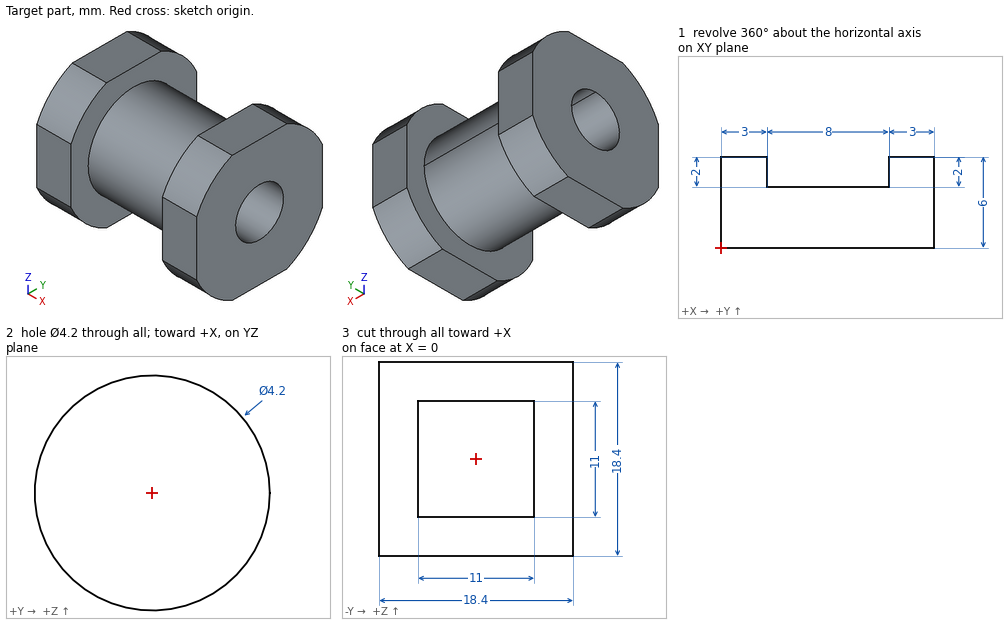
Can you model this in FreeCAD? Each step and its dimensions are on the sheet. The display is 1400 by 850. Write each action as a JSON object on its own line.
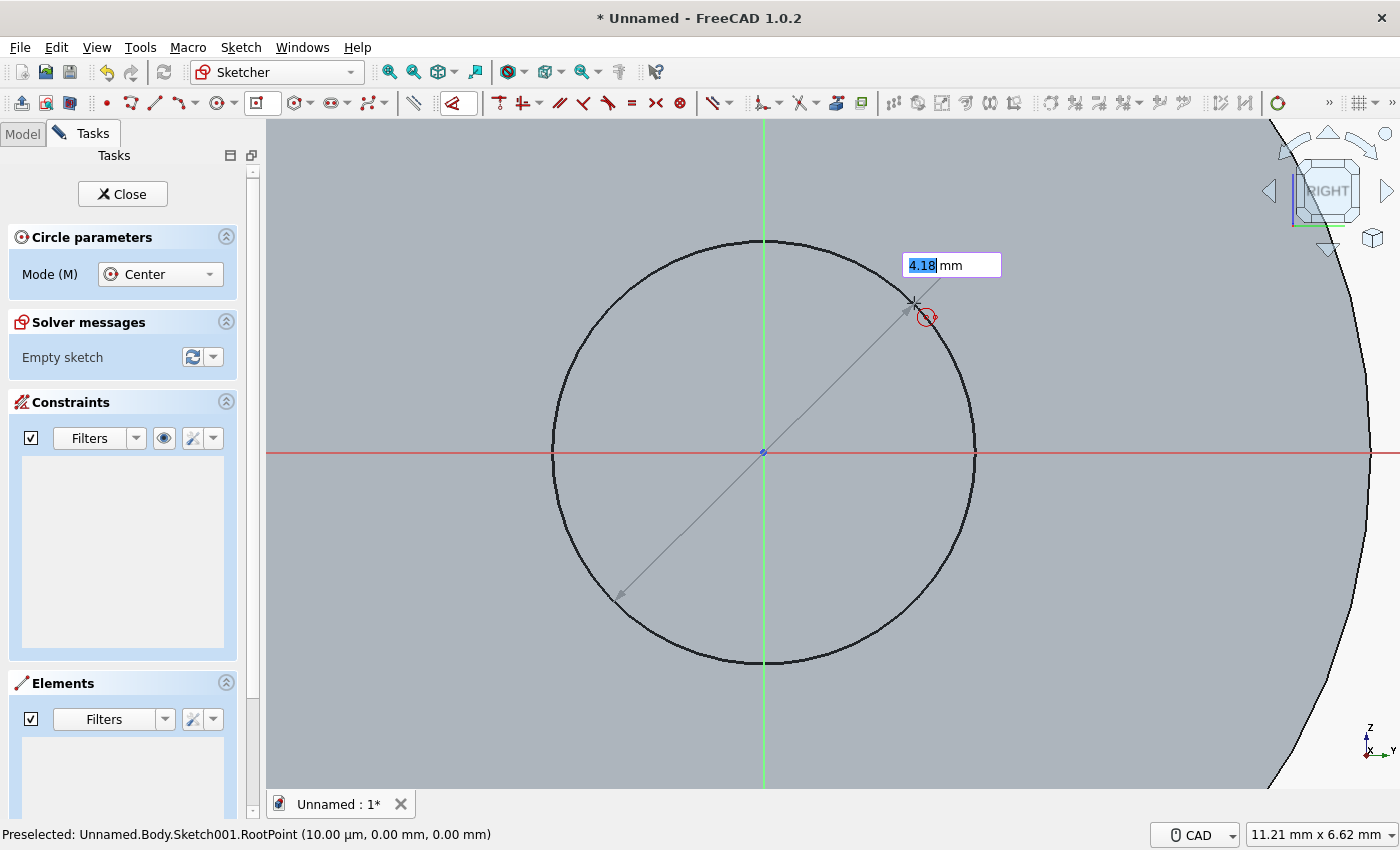
{"action": "type", "text": "4.2"}
{"action": "key", "text": "Return"}
{"action": "key", "text": "Escape"}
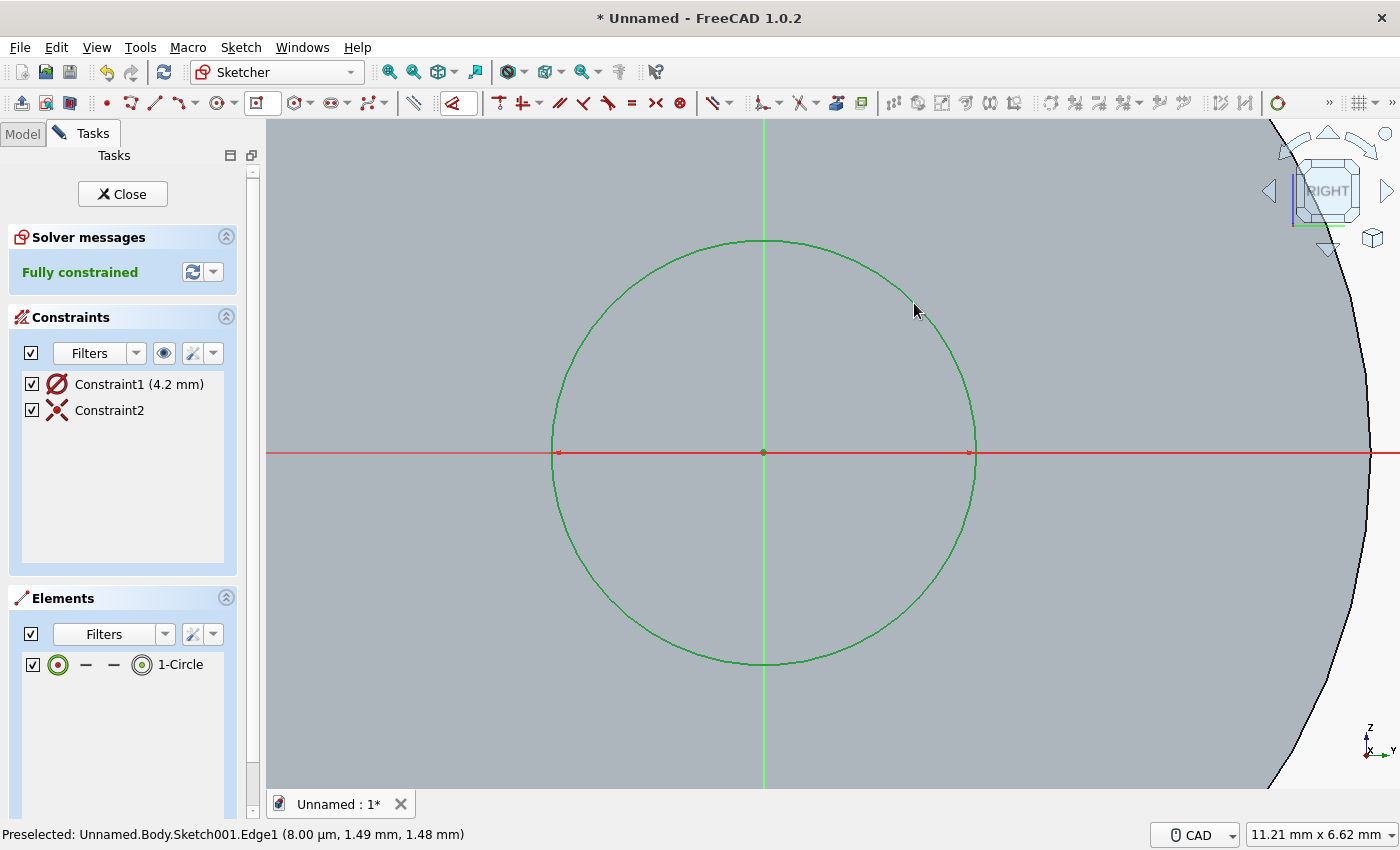
{"action": "left_click", "coordinate": [123, 194]}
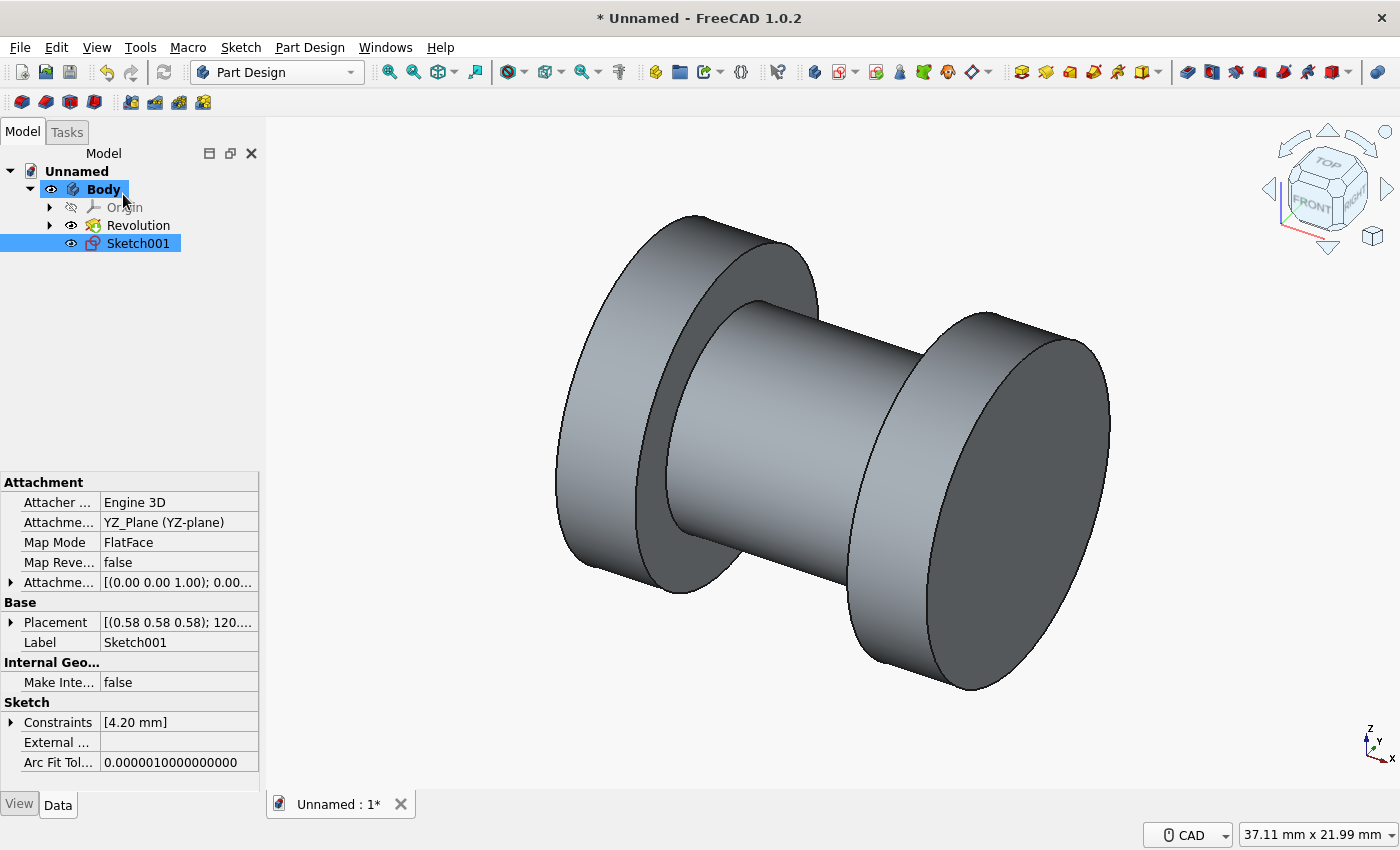
{"action": "left_click", "coordinate": [1212, 72]}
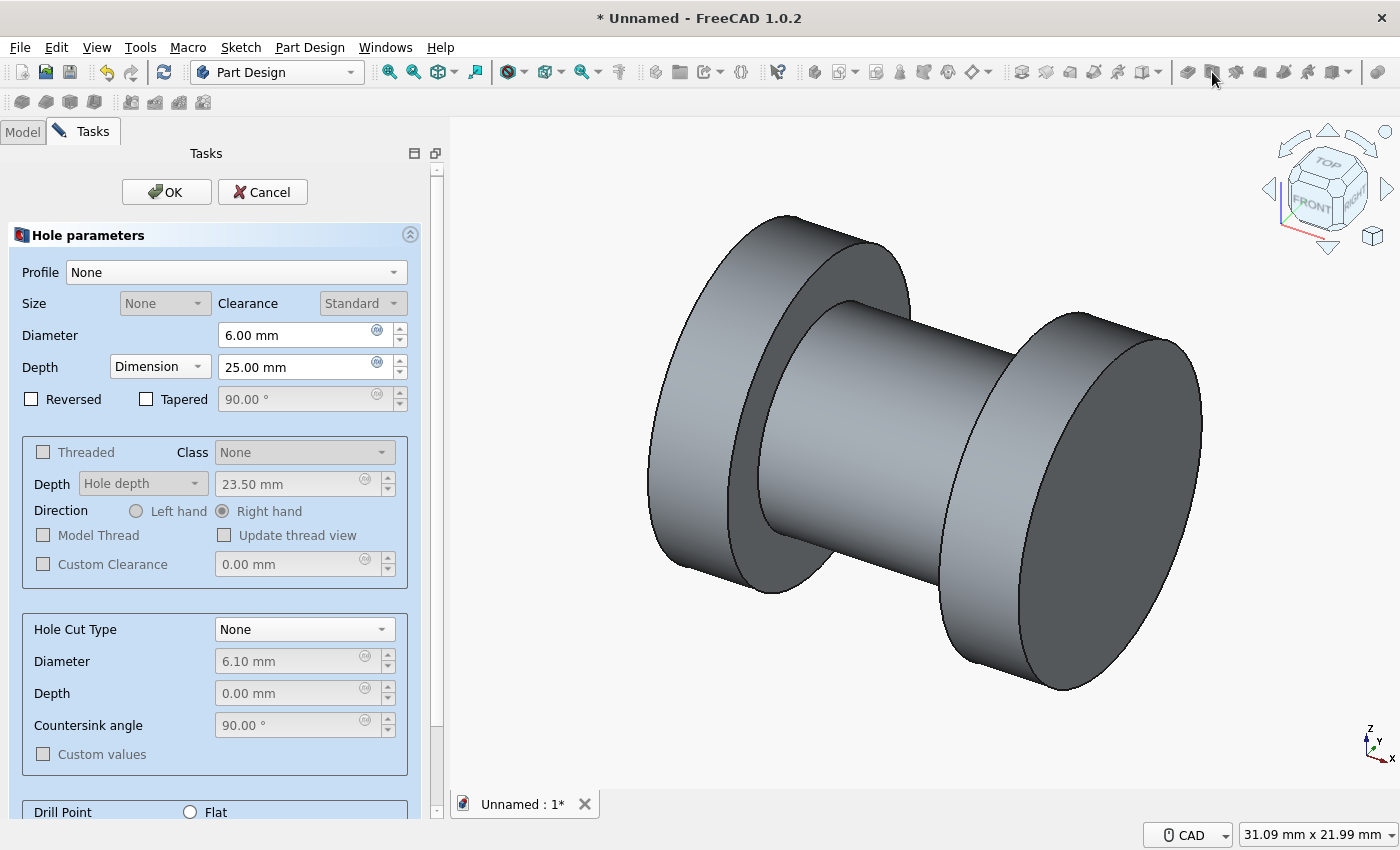
{"action": "triple_click", "coordinate": [305, 335]}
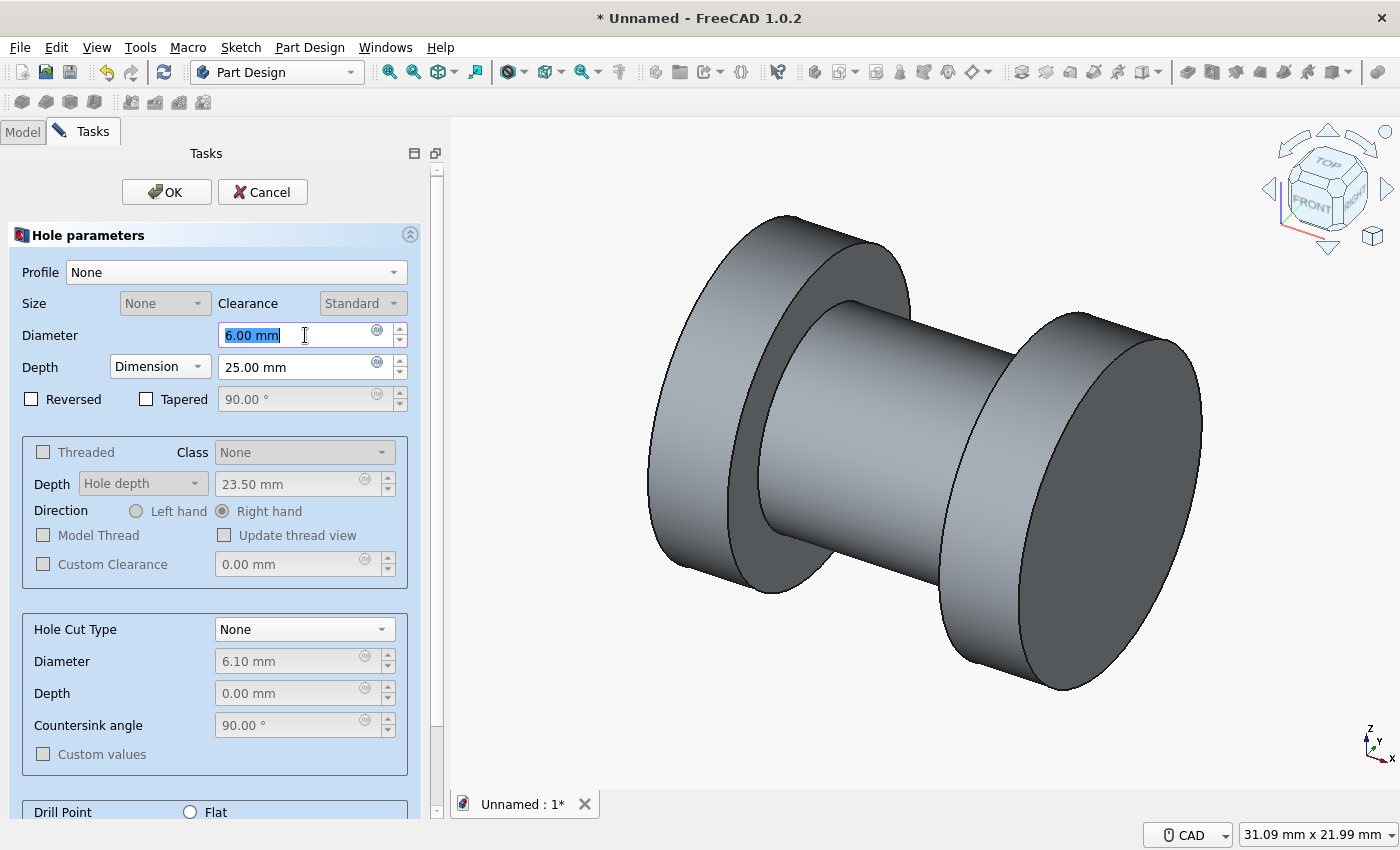
{"action": "type", "text": "4.2"}
{"action": "key", "text": "Tab"}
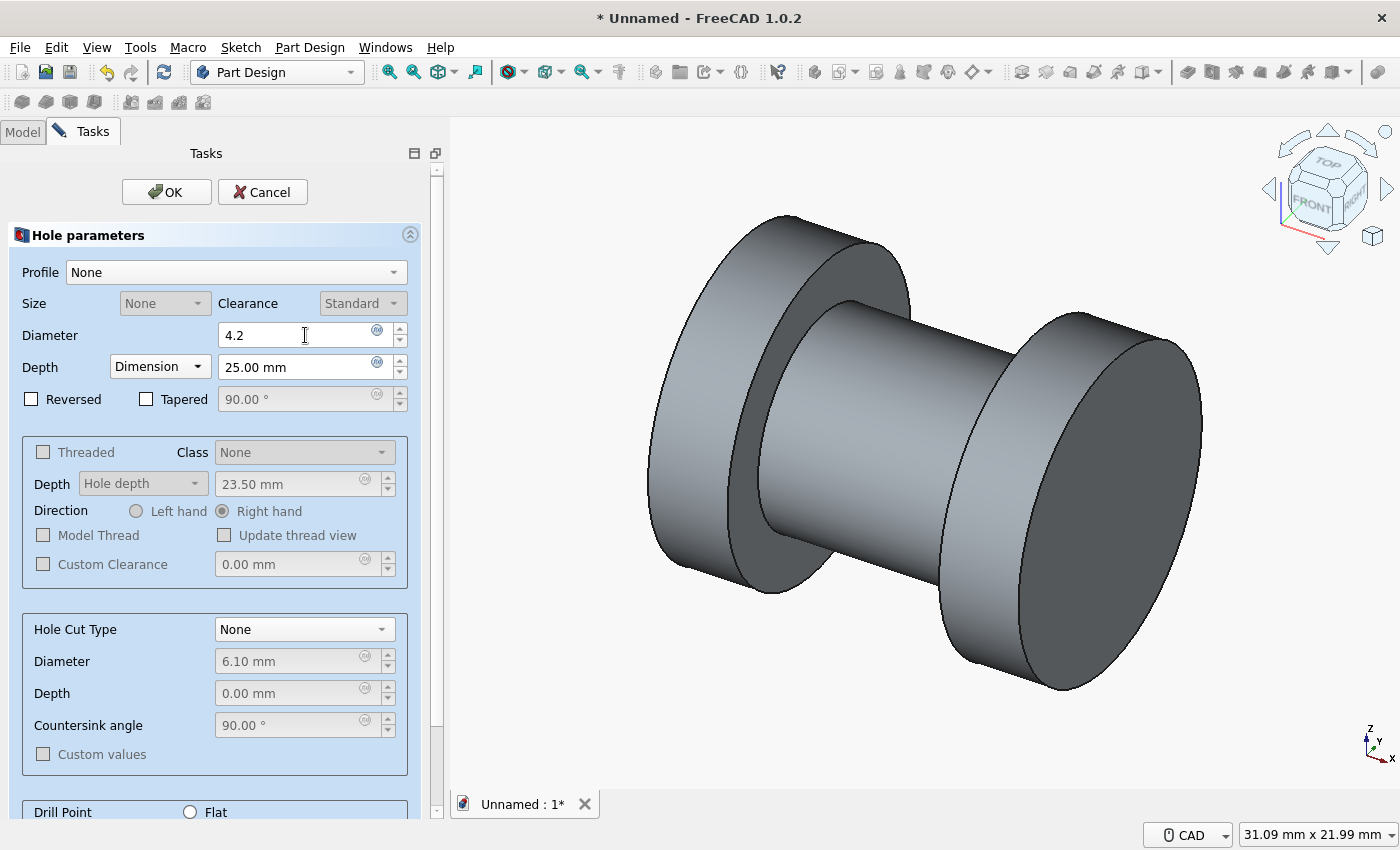
{"action": "left_click", "coordinate": [161, 366]}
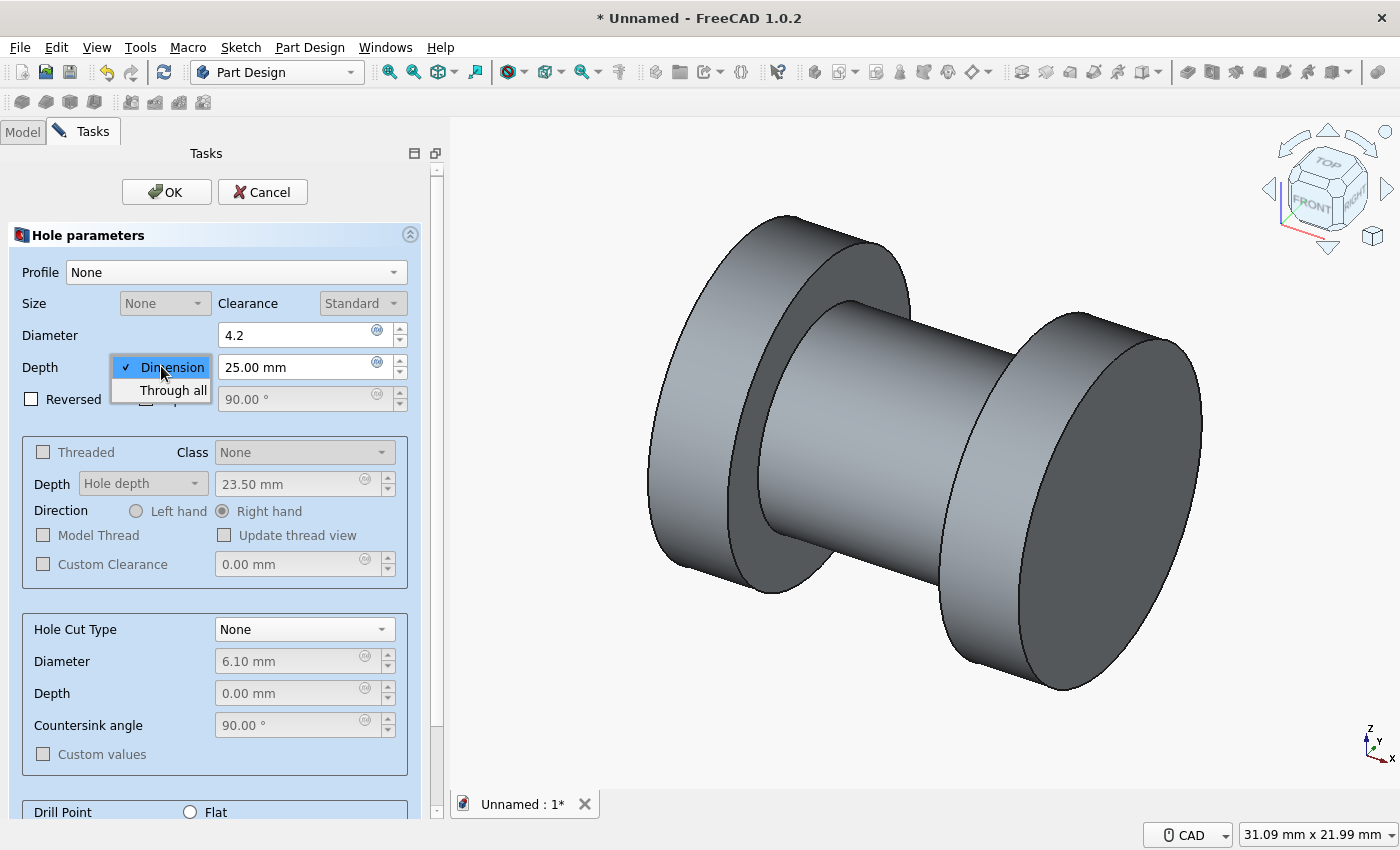
{"action": "left_click", "coordinate": [160, 390]}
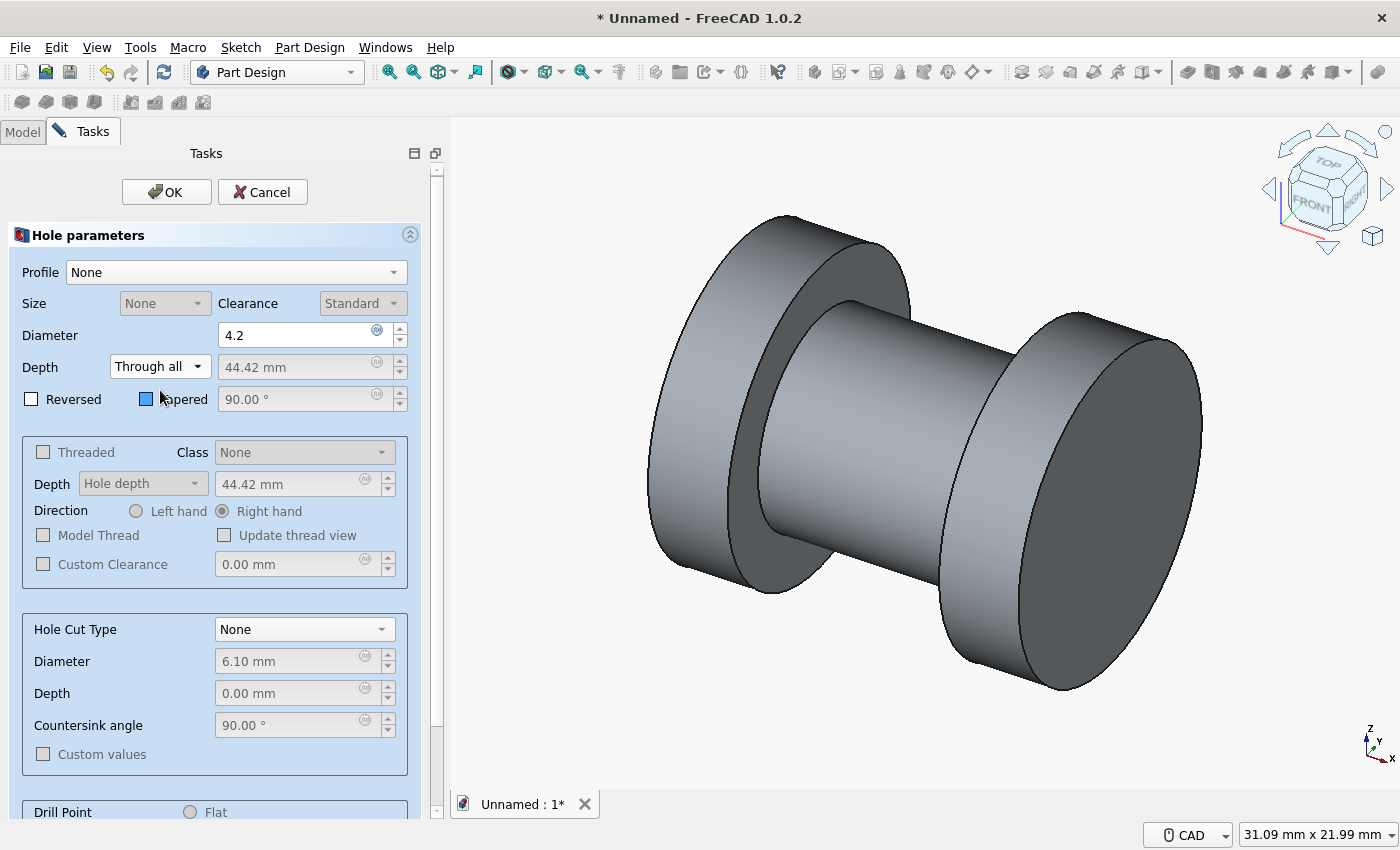
{"action": "left_click", "coordinate": [30, 399]}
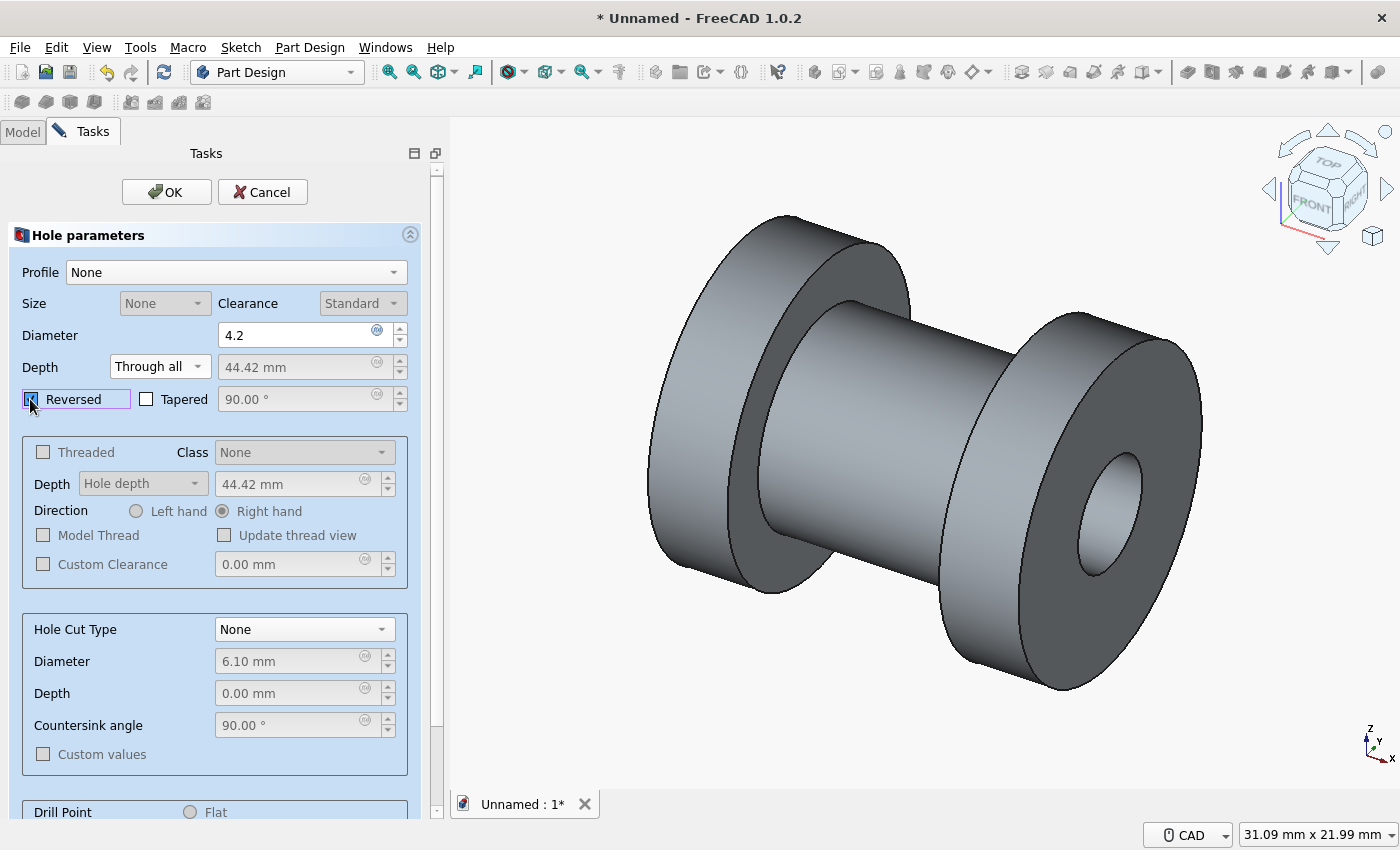
{"action": "left_click", "coordinate": [167, 192]}